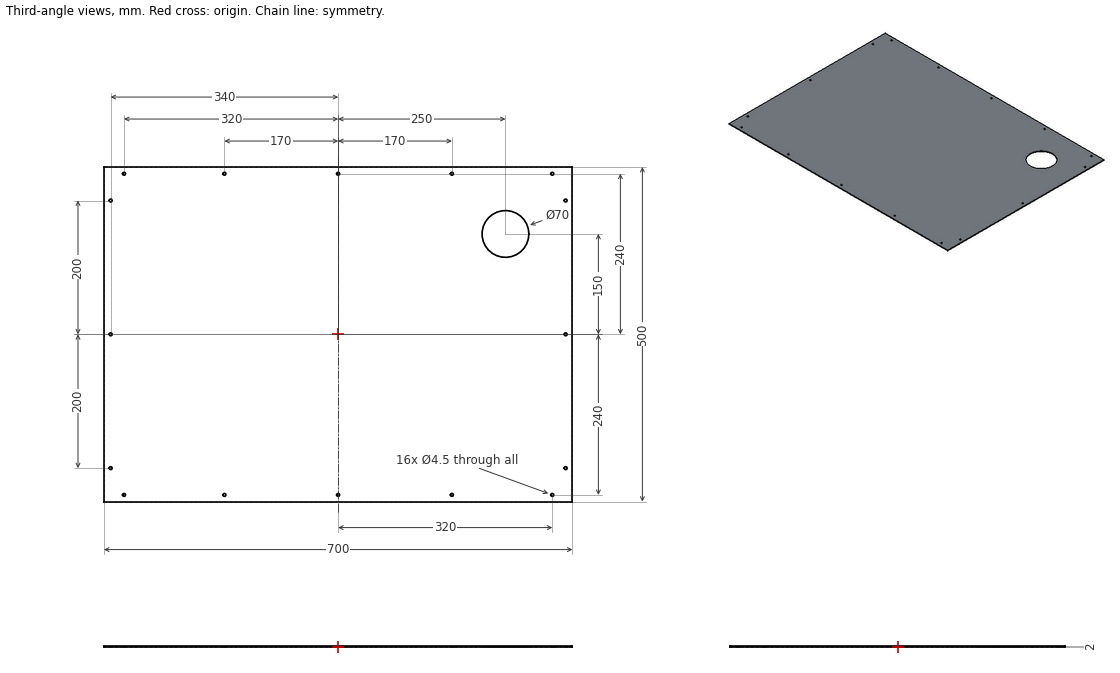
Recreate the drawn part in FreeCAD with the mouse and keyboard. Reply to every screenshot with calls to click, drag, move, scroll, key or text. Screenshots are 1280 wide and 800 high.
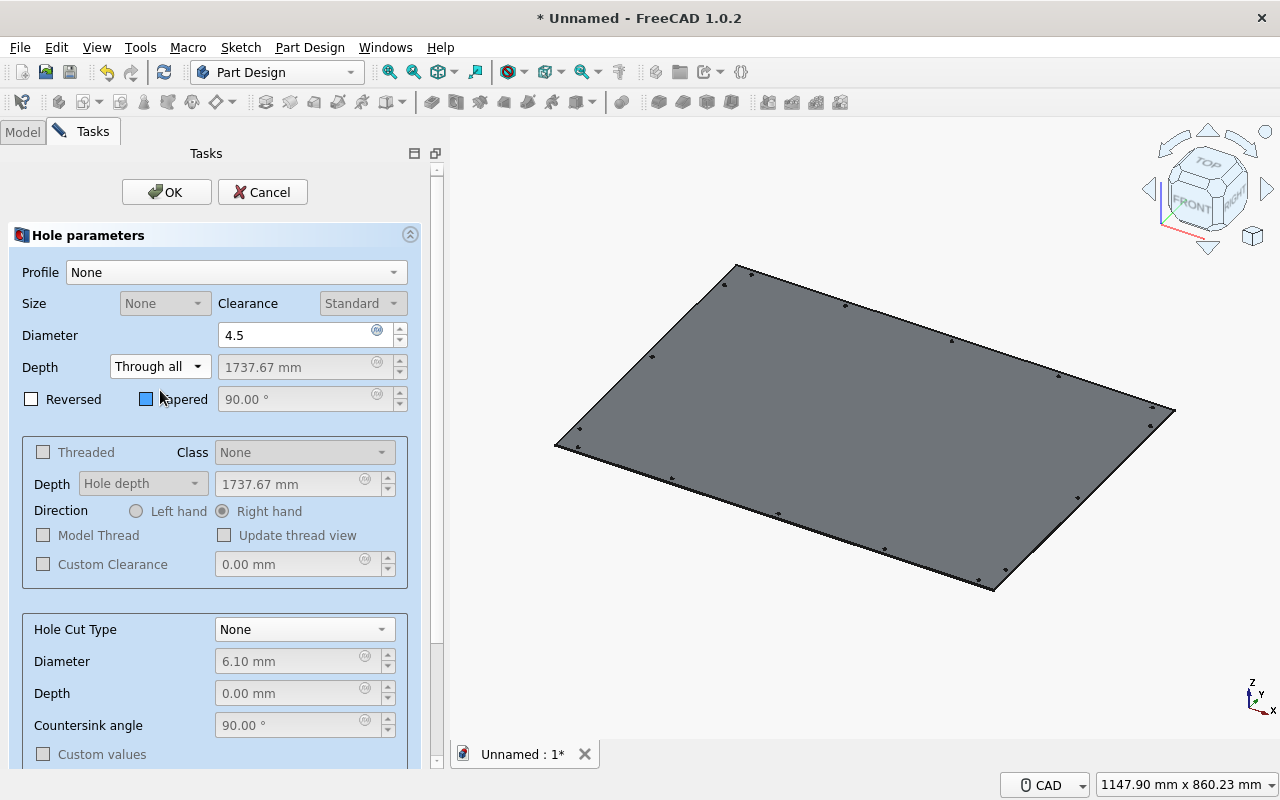
click(167, 192)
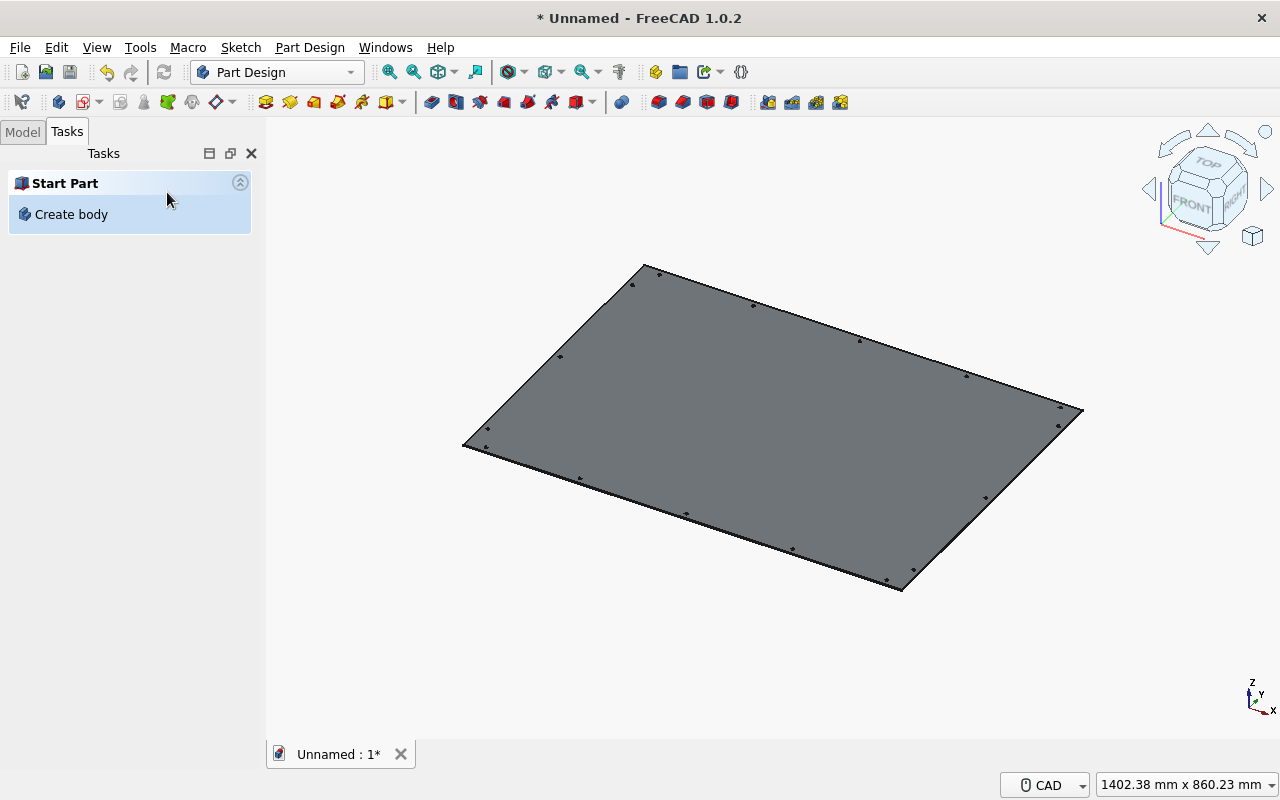
click(836, 447)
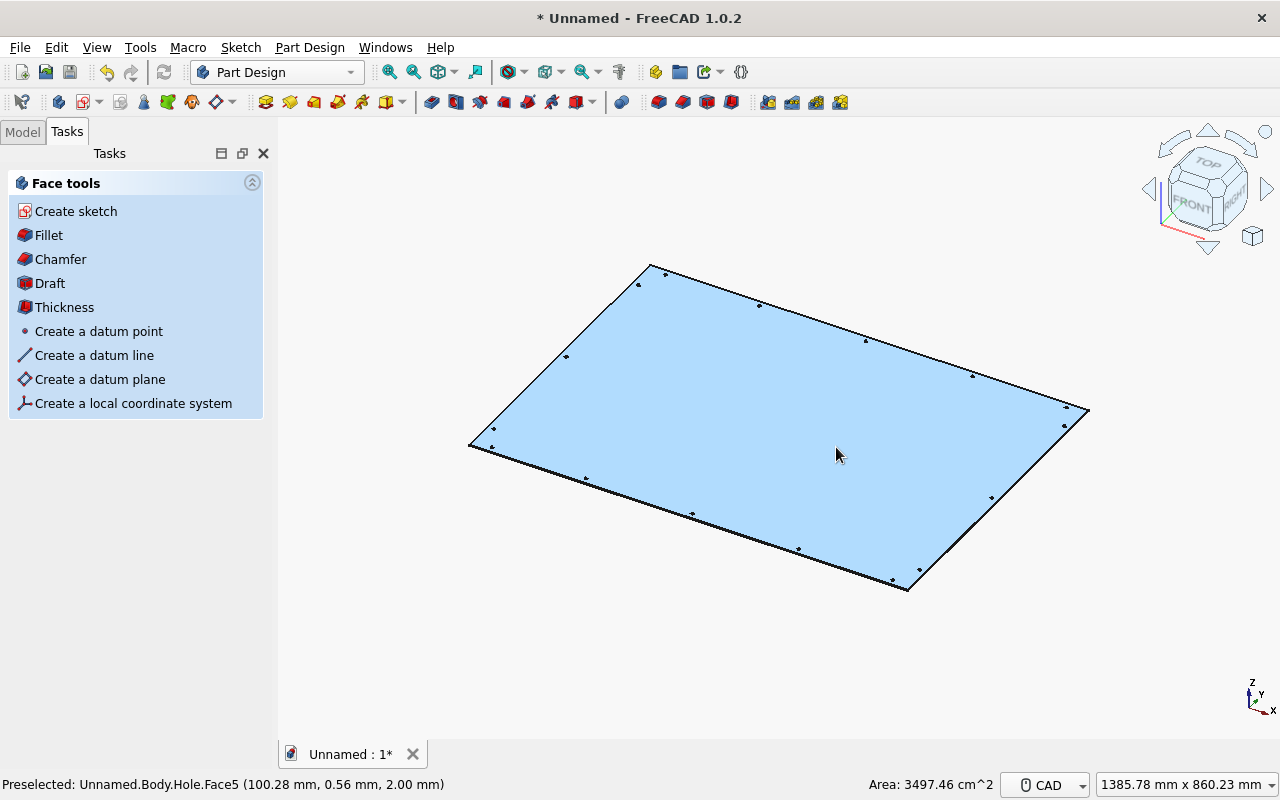
click(84, 102)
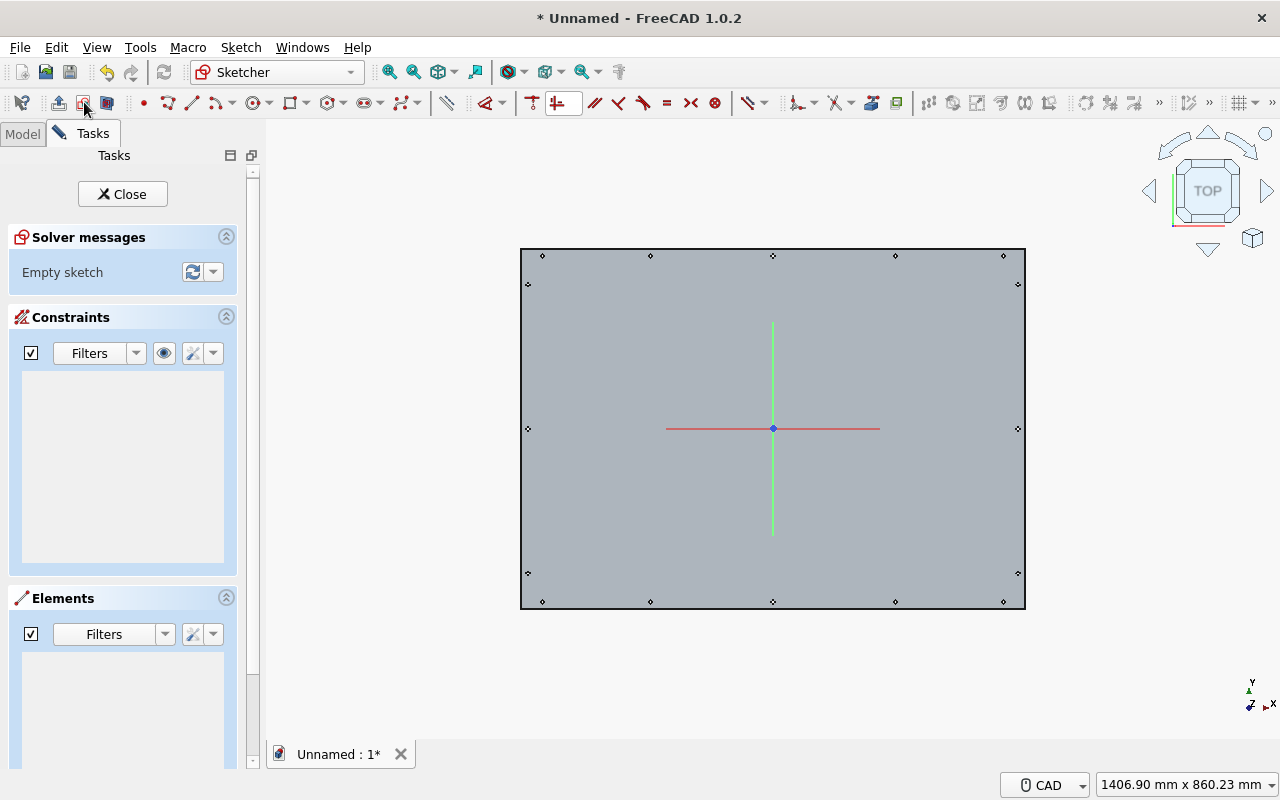
scroll(992, 304, up, 10)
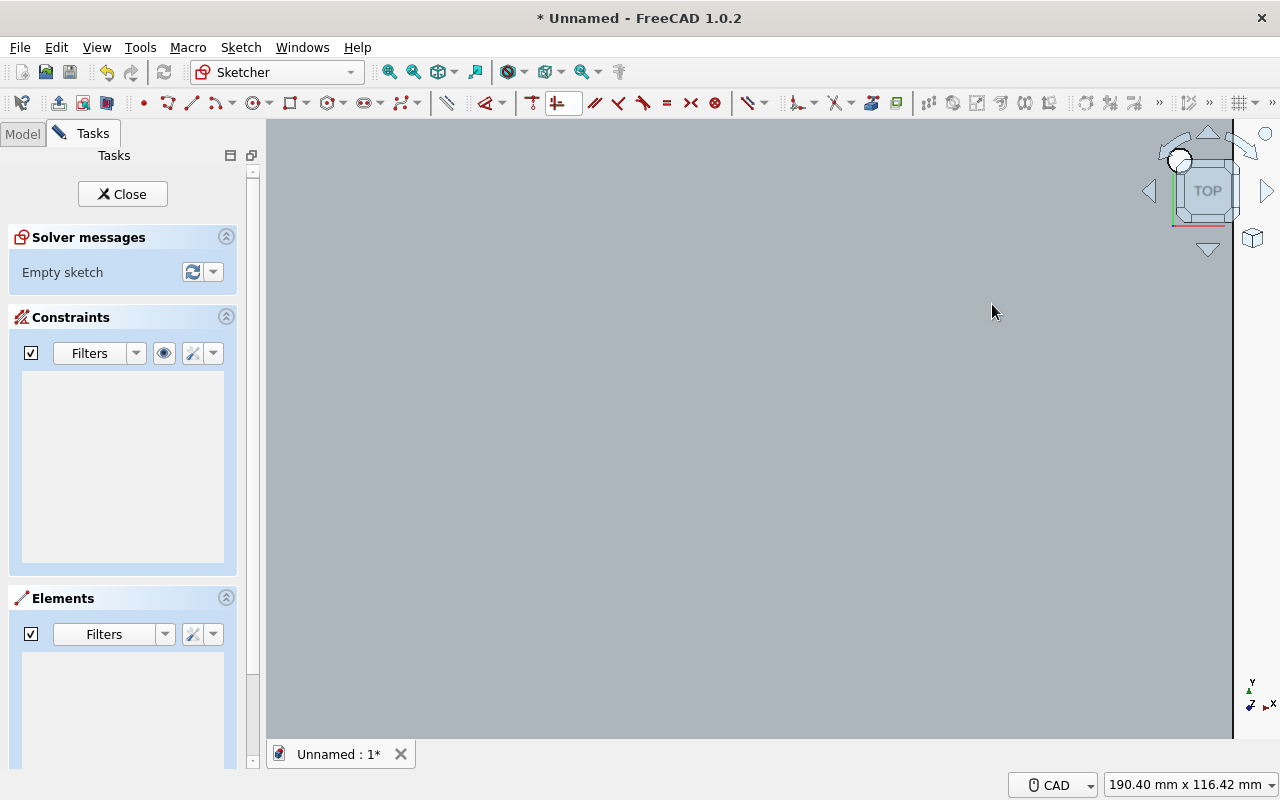
click(254, 104)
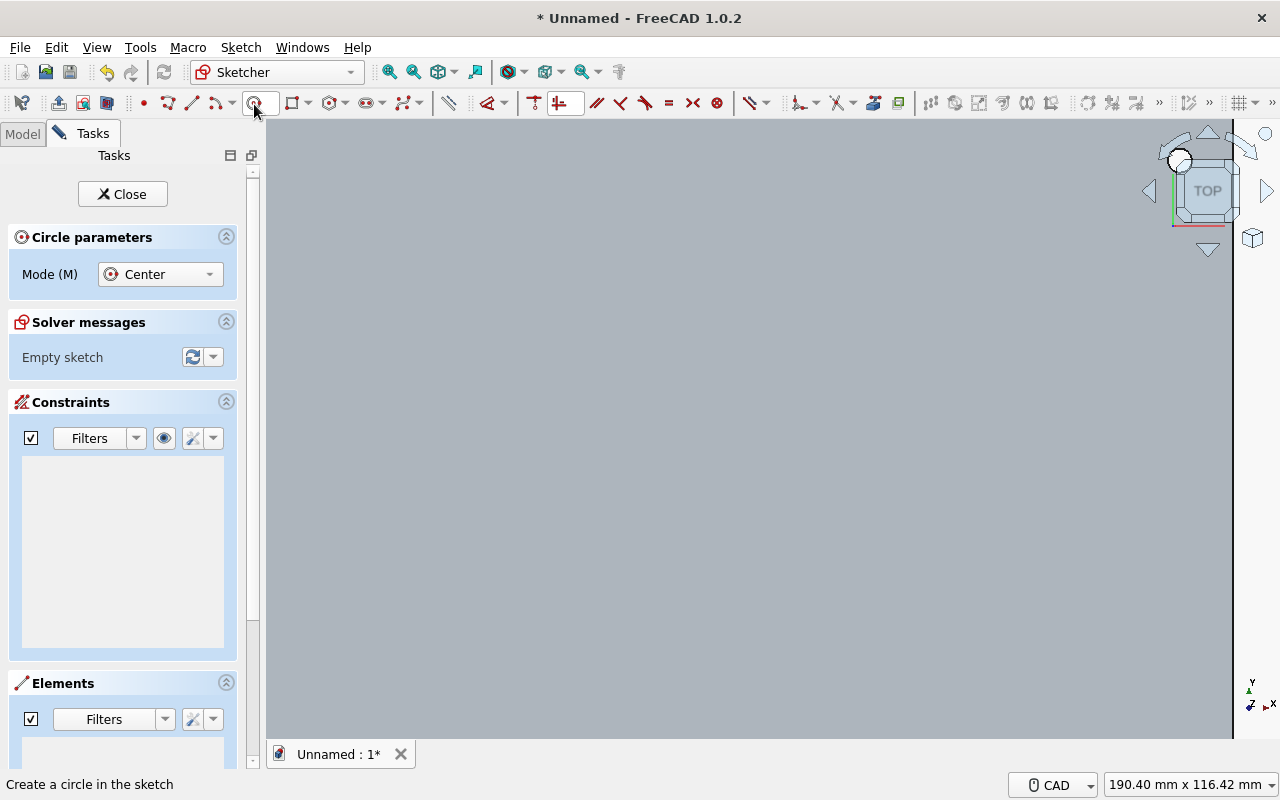
click(701, 427)
move(832, 295)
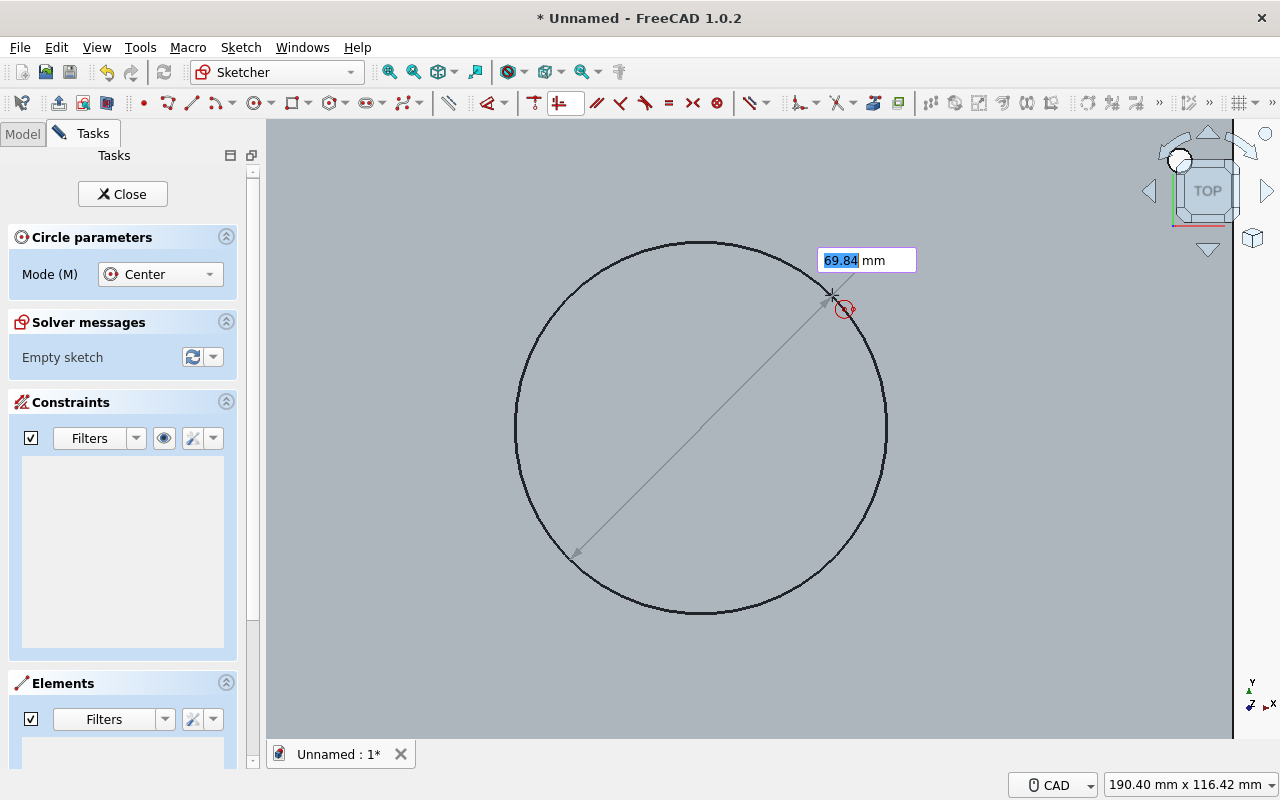
text(70)
key(Return)
key(Escape)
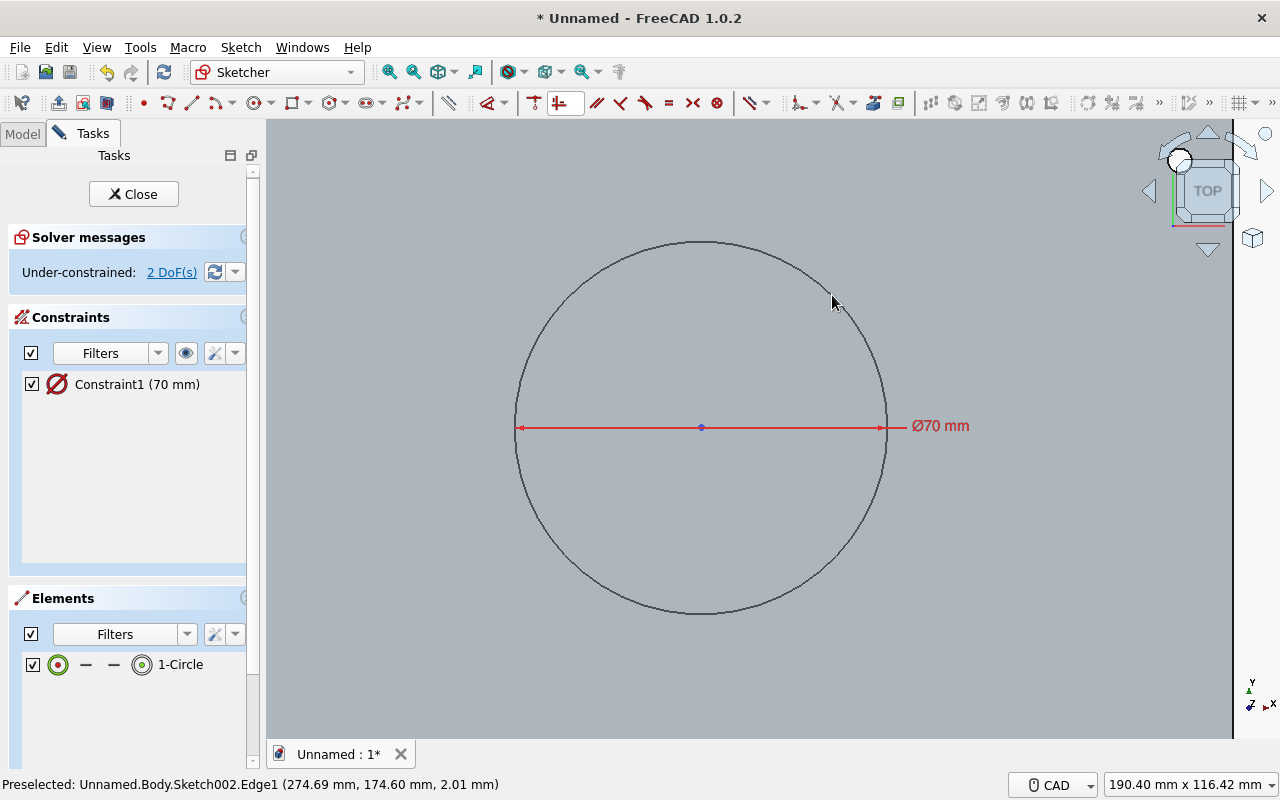
key(d)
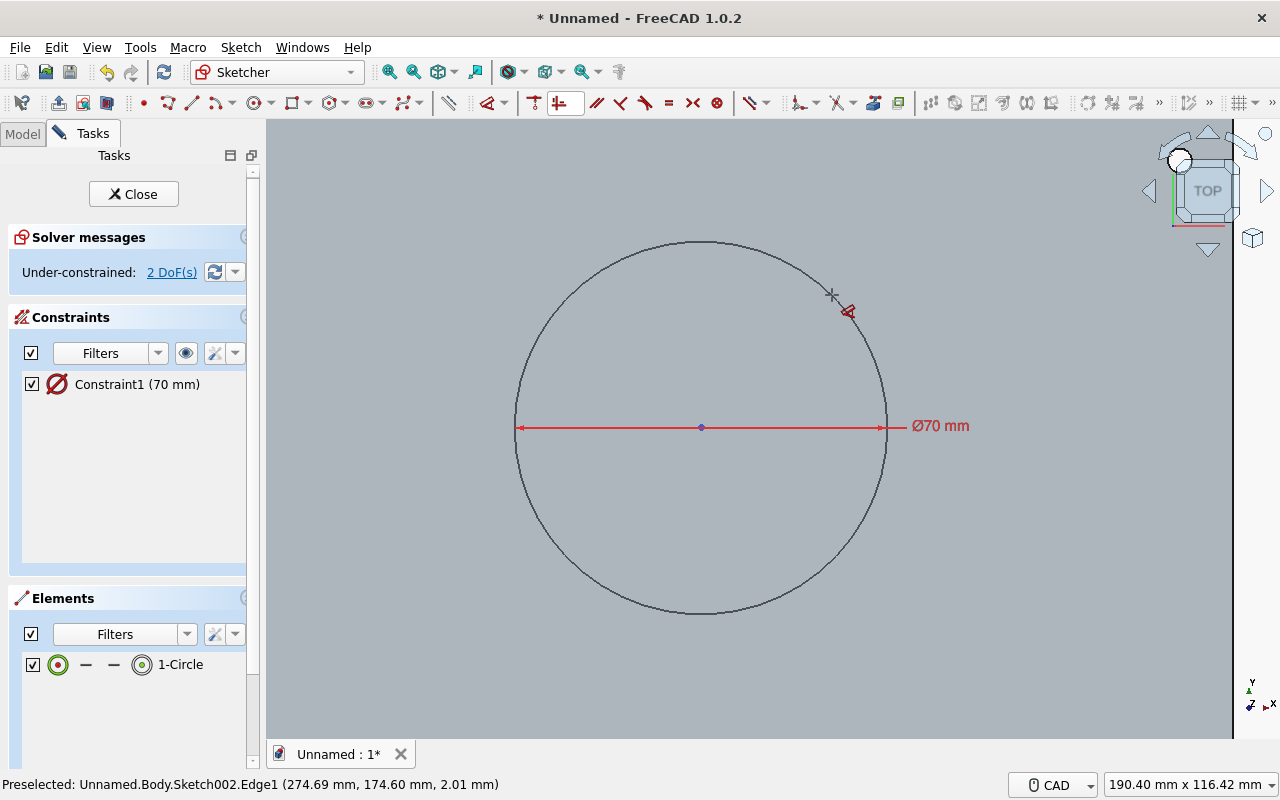
click(701, 428)
click(498, 394)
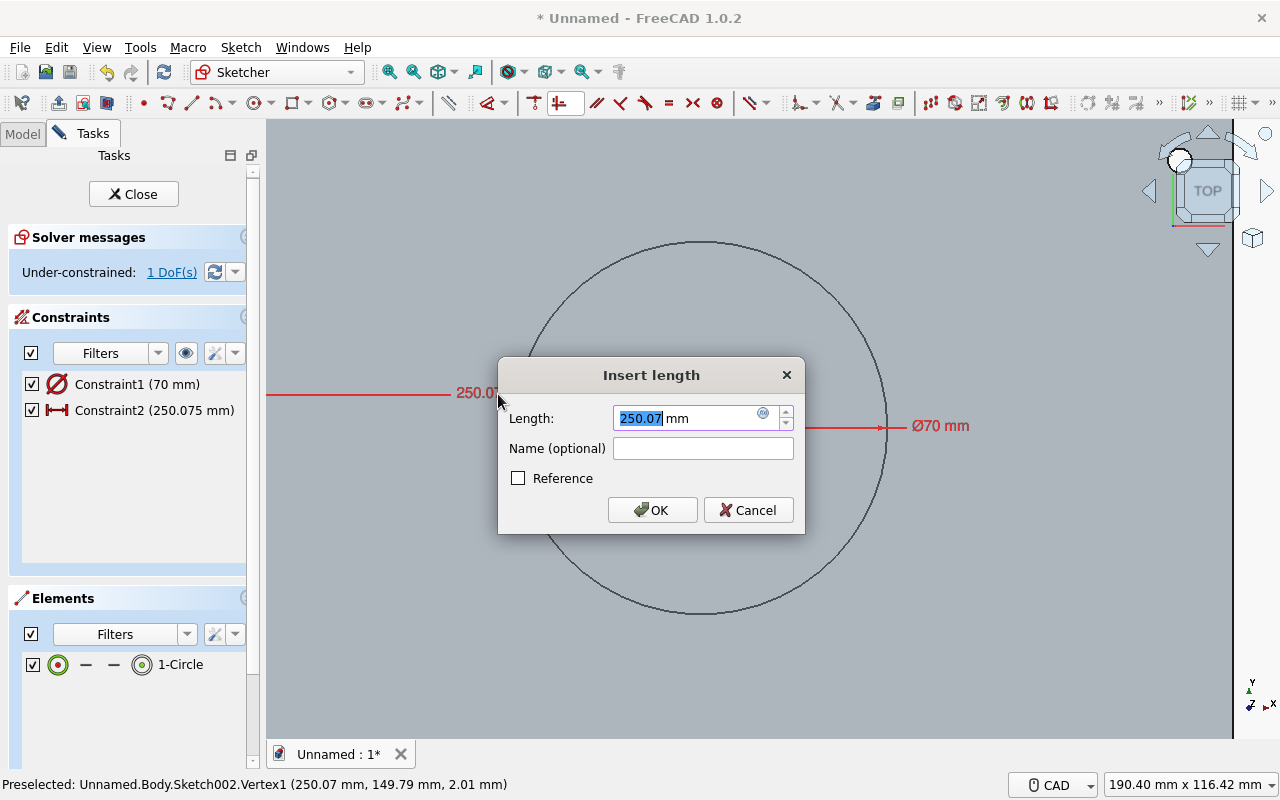
text(250)
key(Return)